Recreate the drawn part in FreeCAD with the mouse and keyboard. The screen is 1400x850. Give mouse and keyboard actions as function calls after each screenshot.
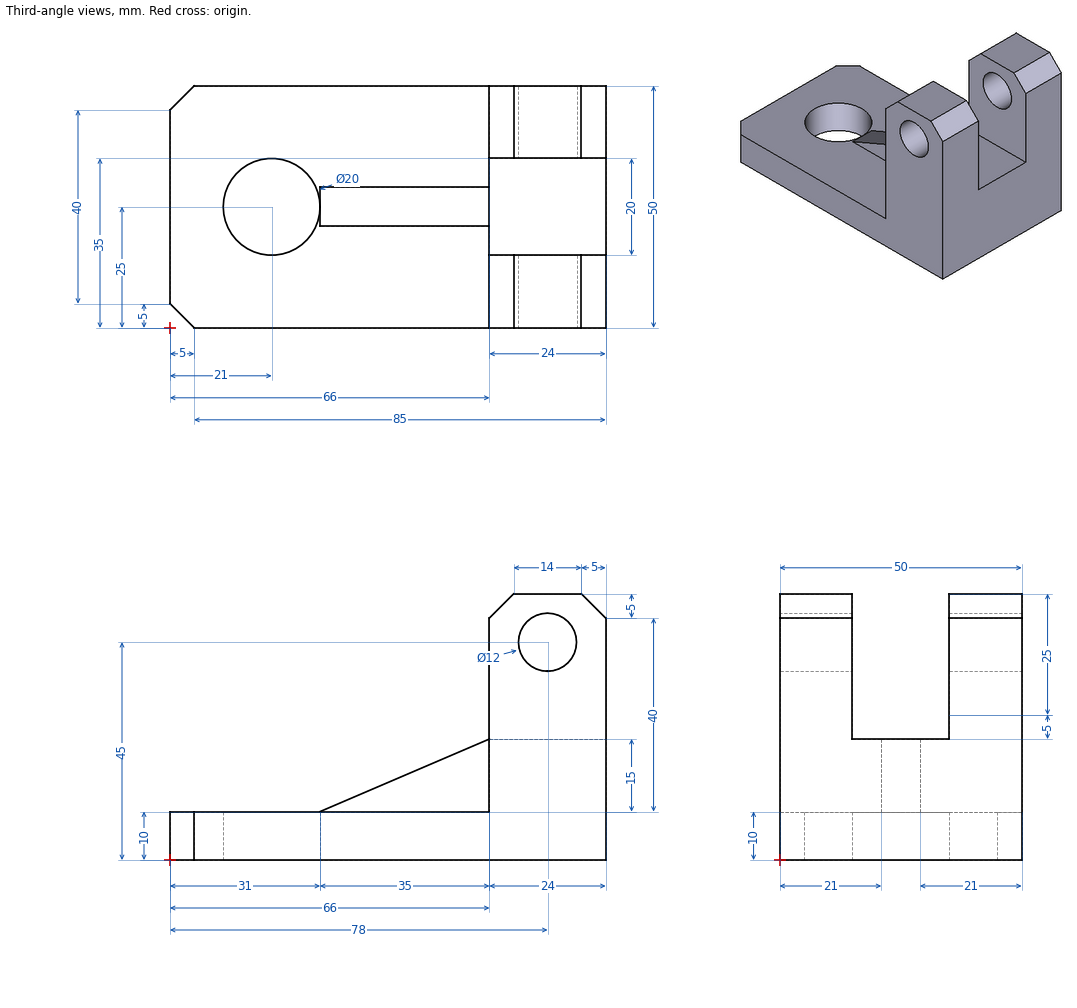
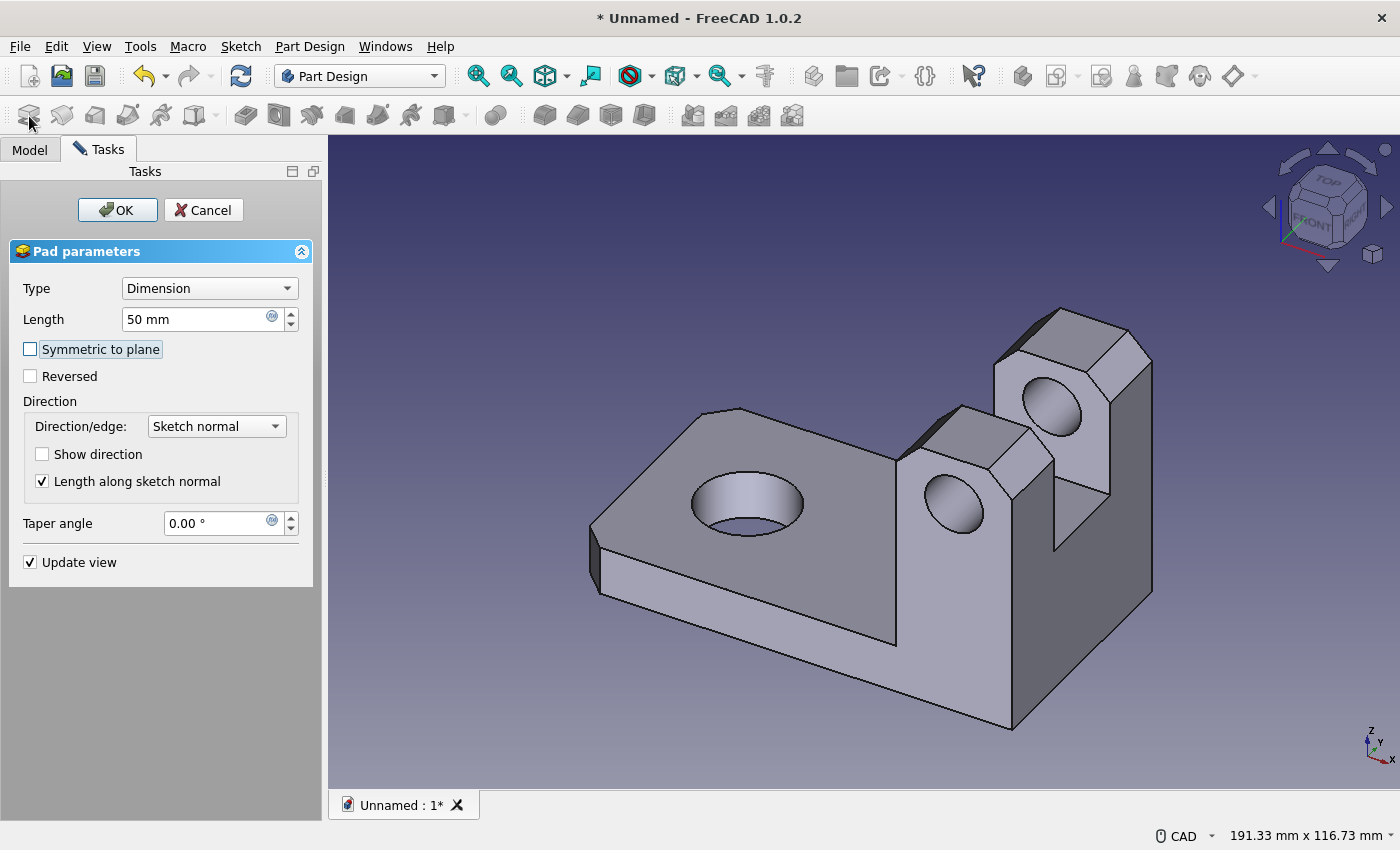
click(31, 376)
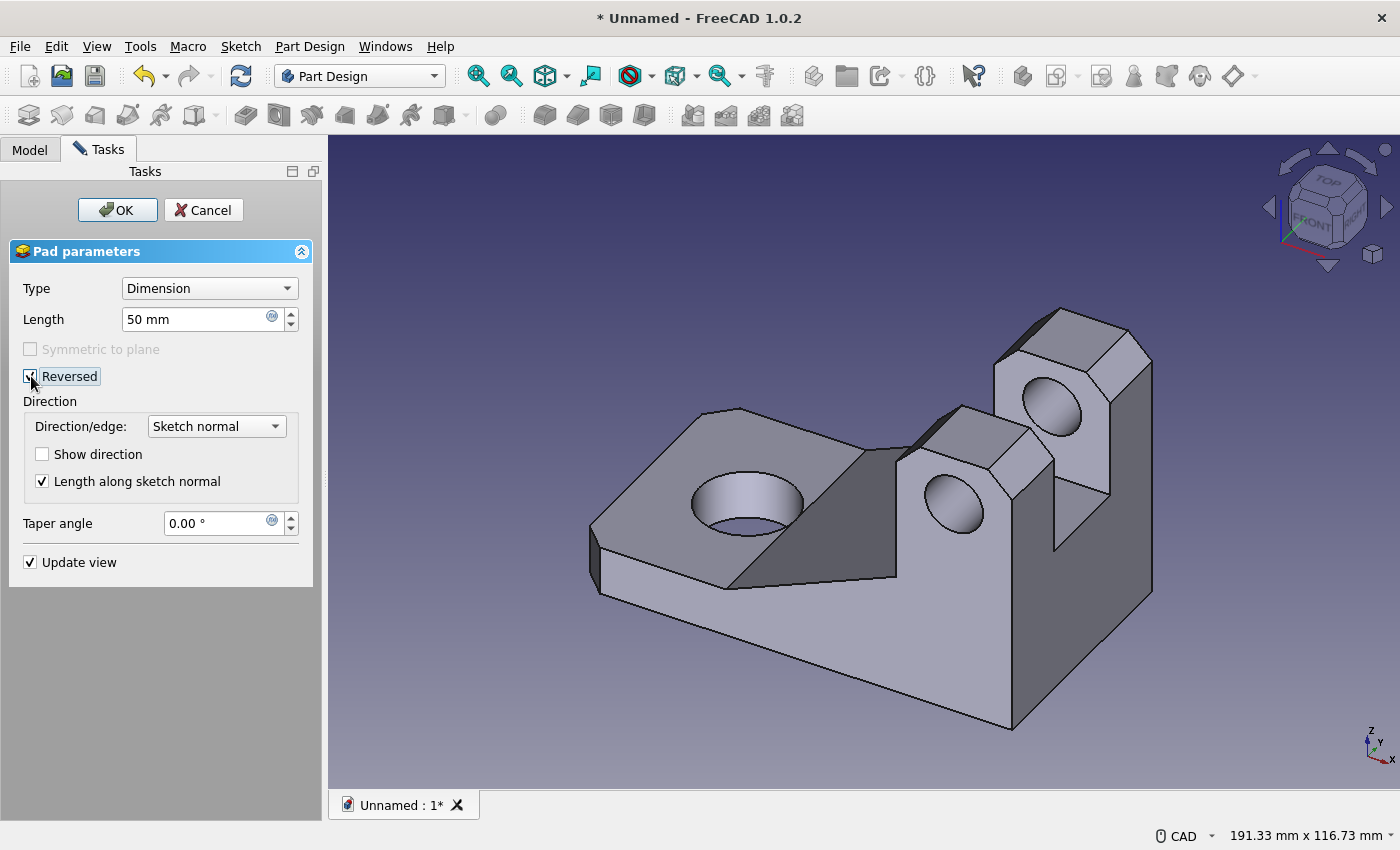
click(118, 210)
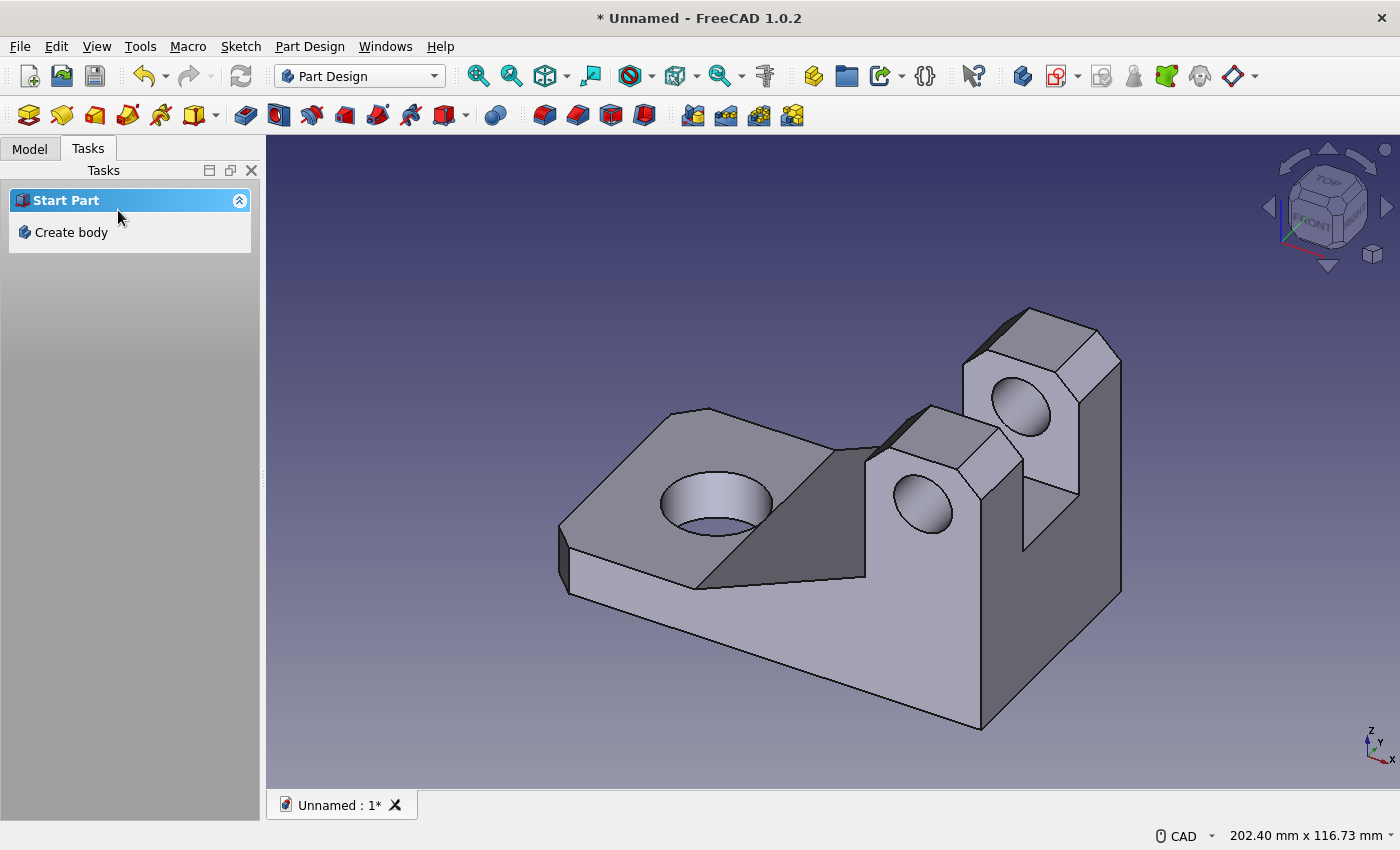
click(893, 646)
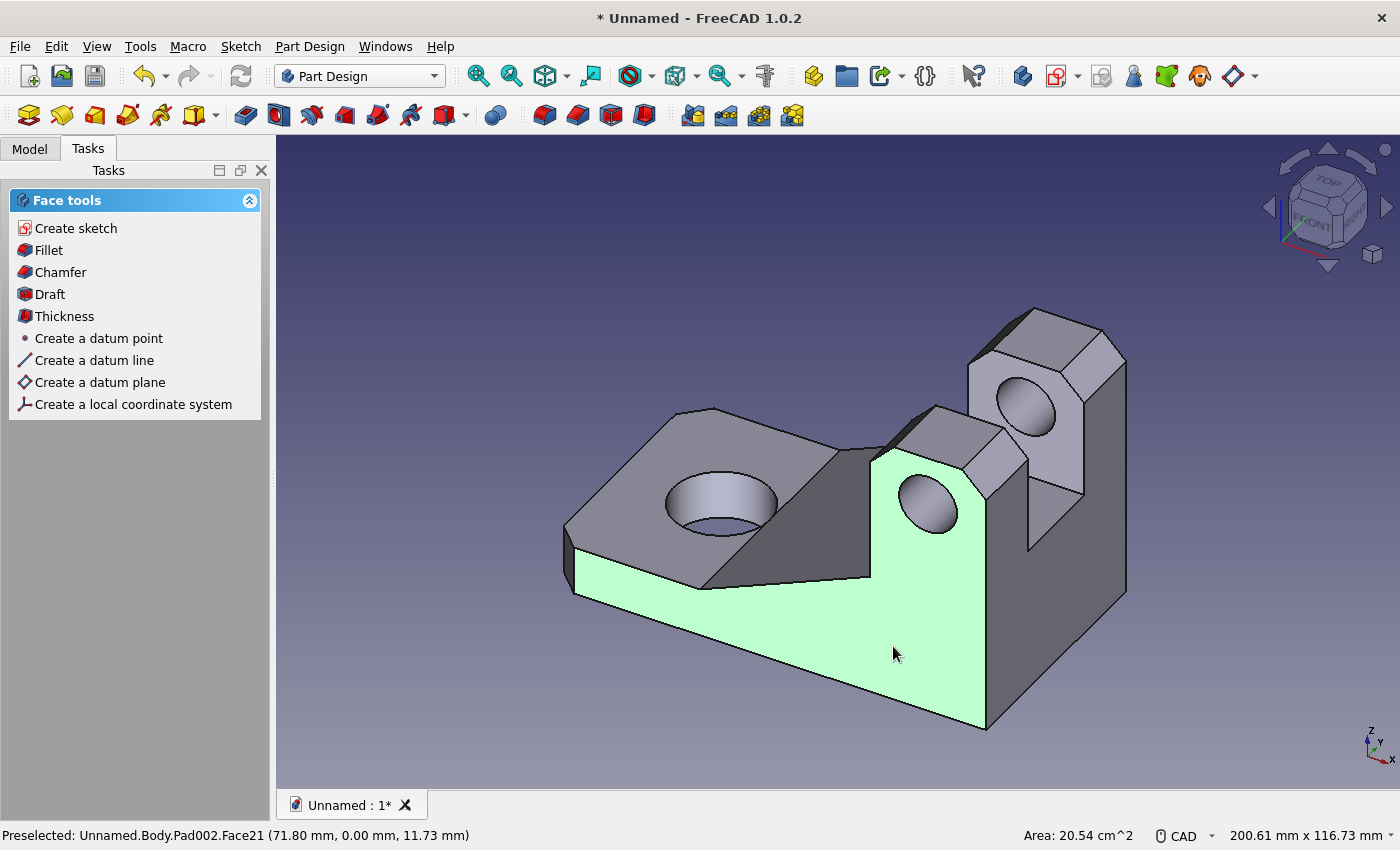
click(1056, 76)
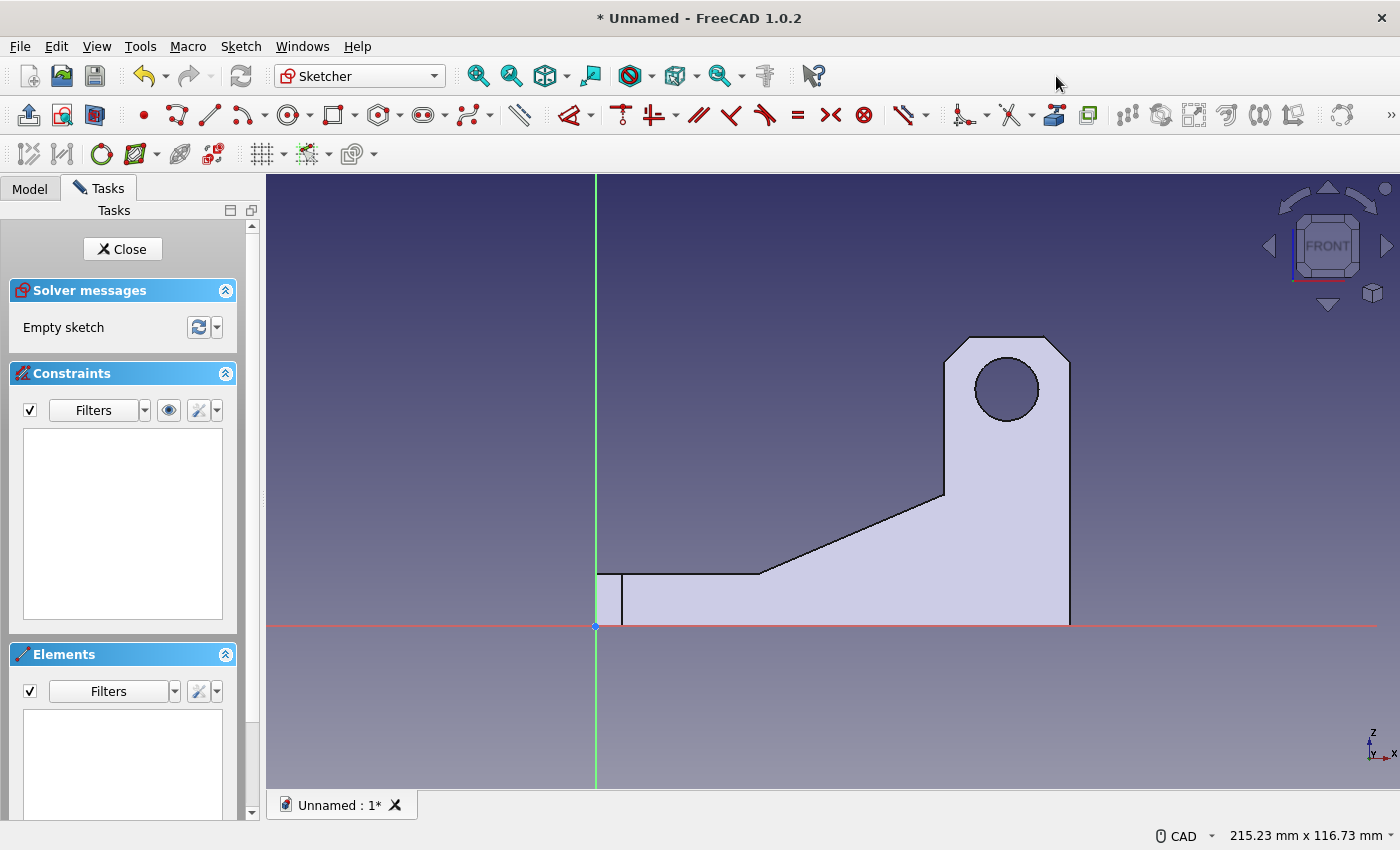
scroll(776, 657, up, 3)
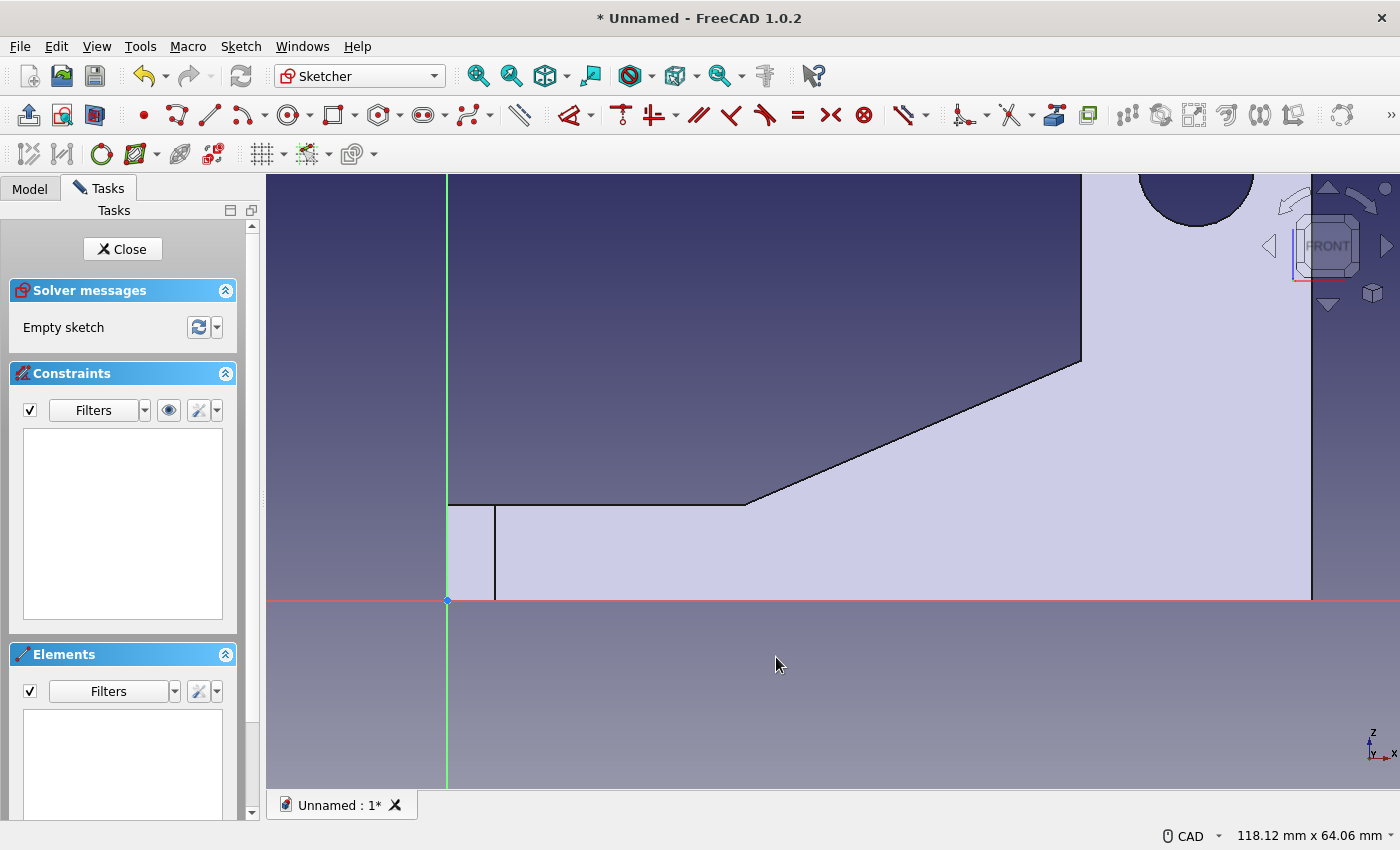
click(177, 116)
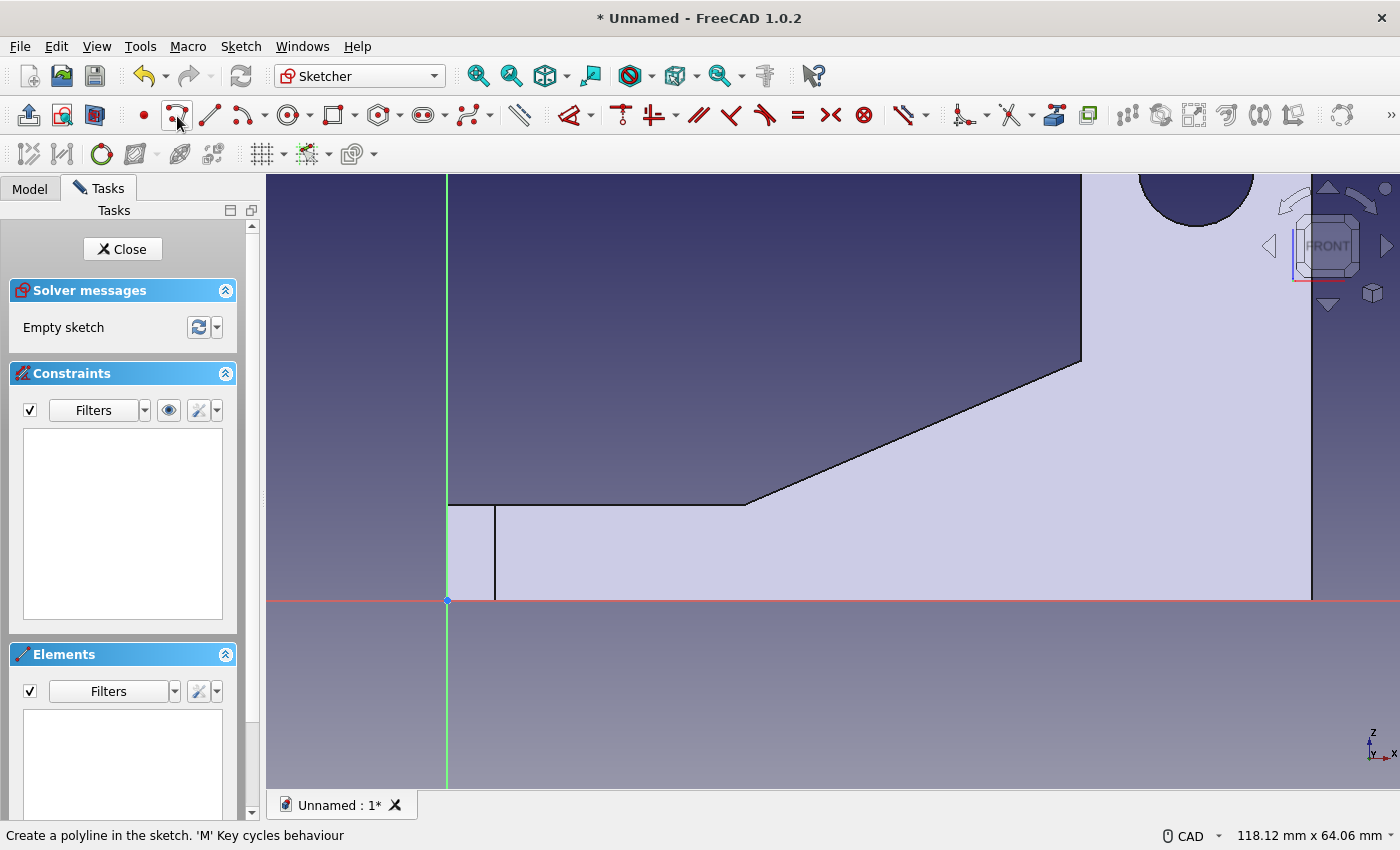
click(745, 505)
click(1081, 505)
click(1081, 361)
click(745, 506)
key(Escape)
key(Escape)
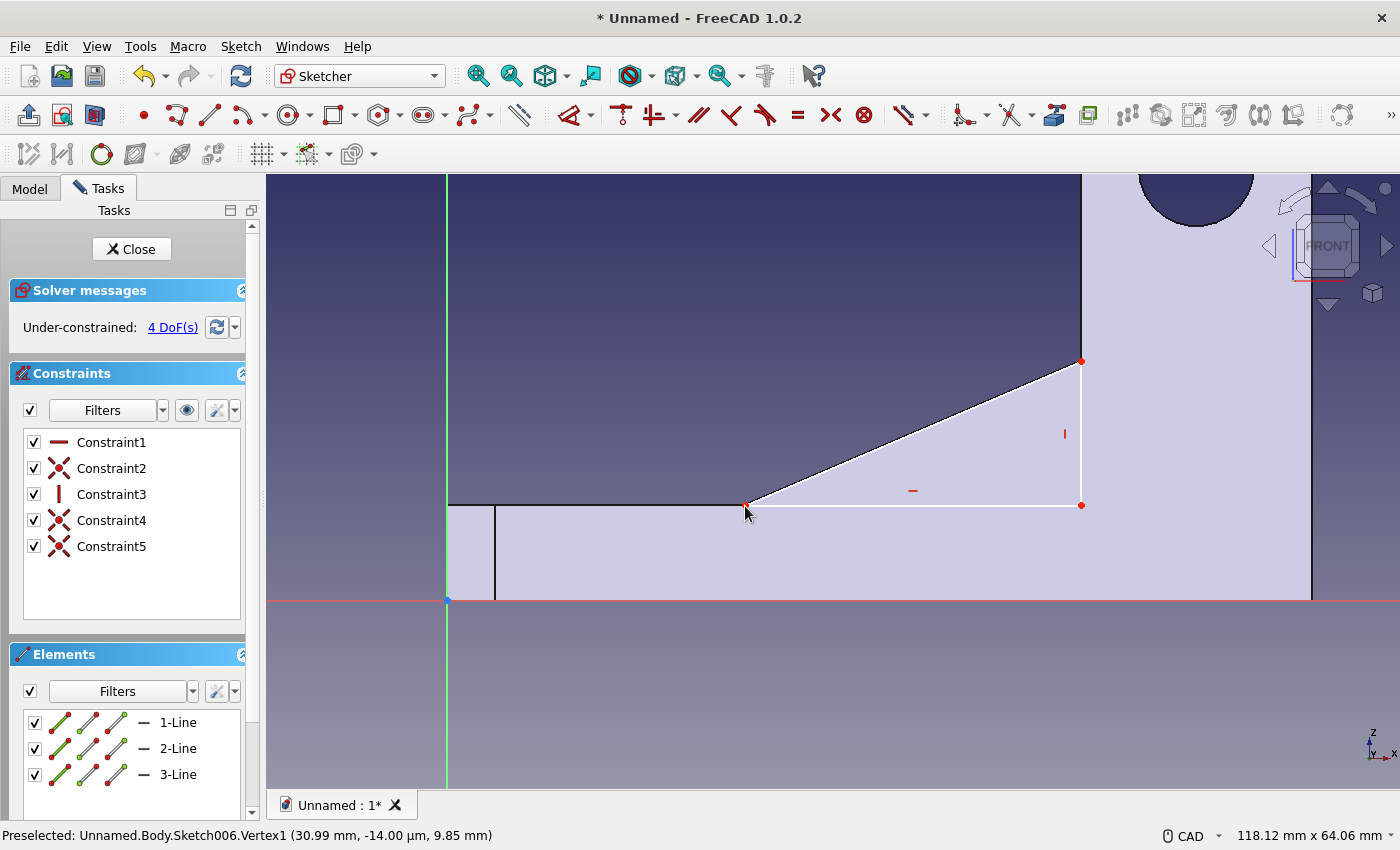
click(568, 116)